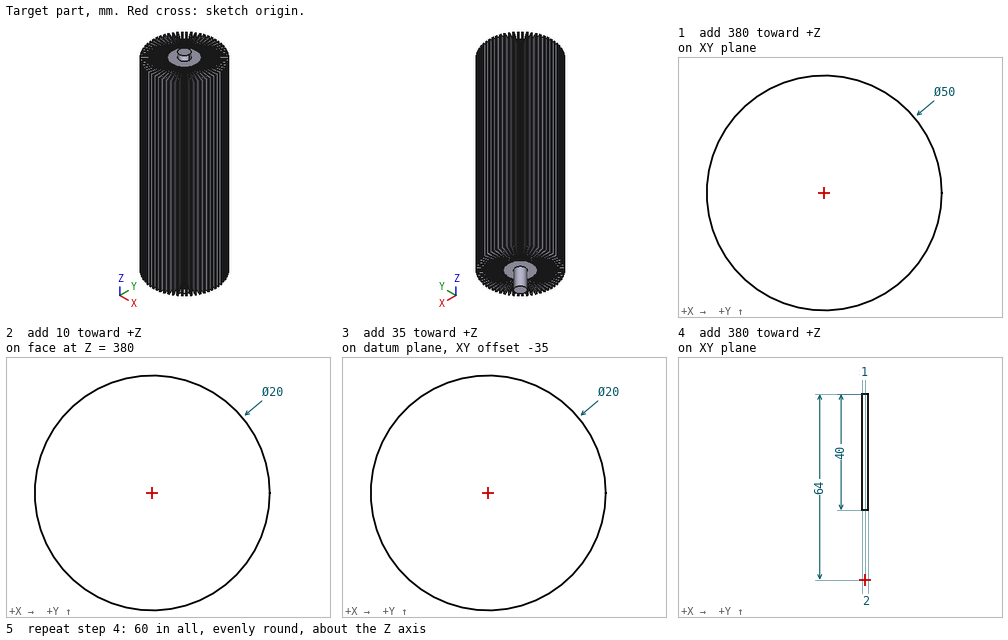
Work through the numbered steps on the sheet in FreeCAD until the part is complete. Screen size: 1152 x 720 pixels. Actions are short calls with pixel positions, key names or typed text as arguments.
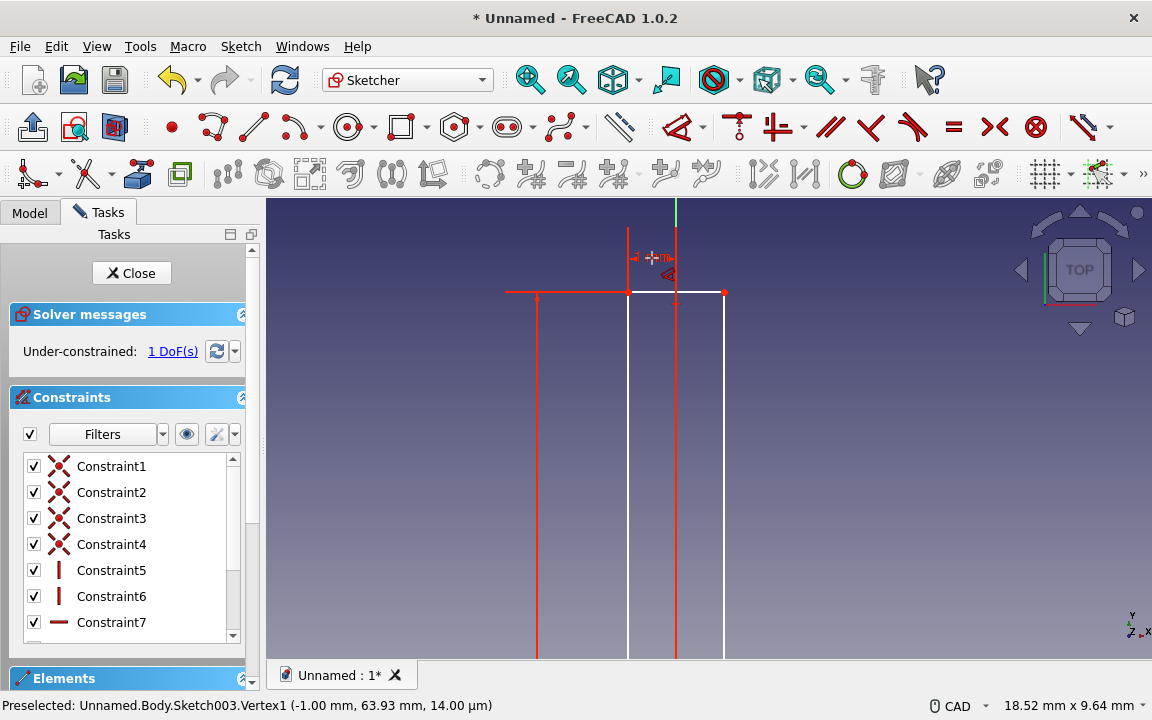
scroll(637, 290, down, 12)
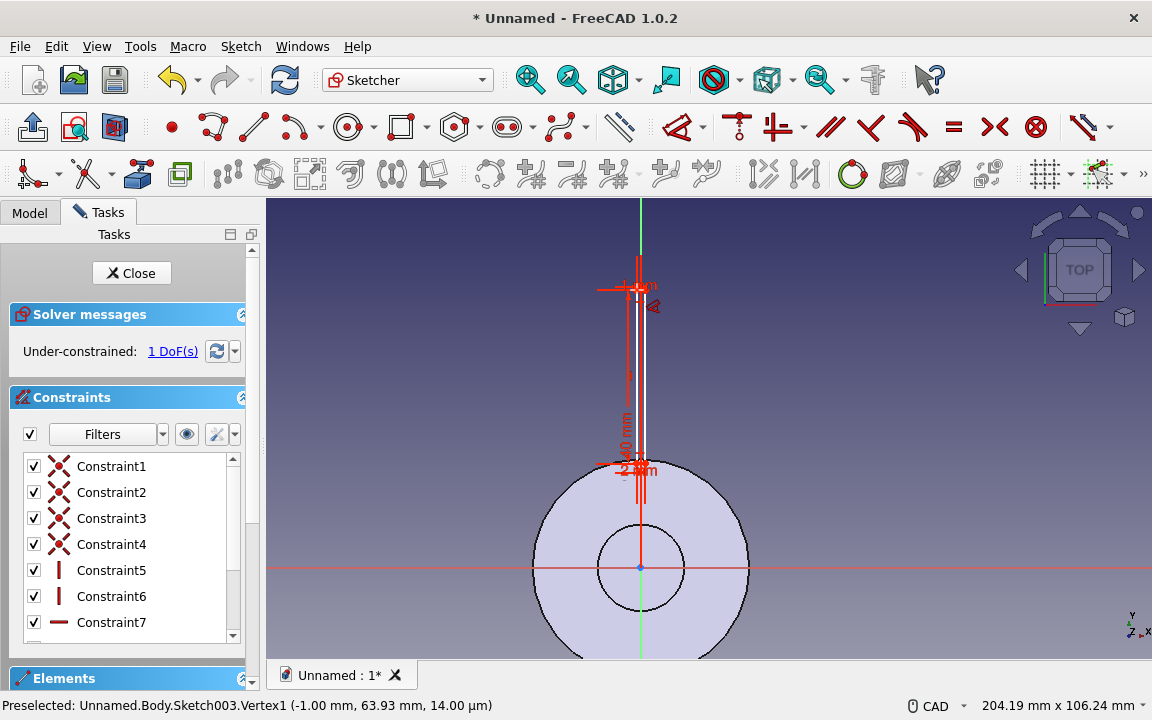
scroll(637, 290, up, 2)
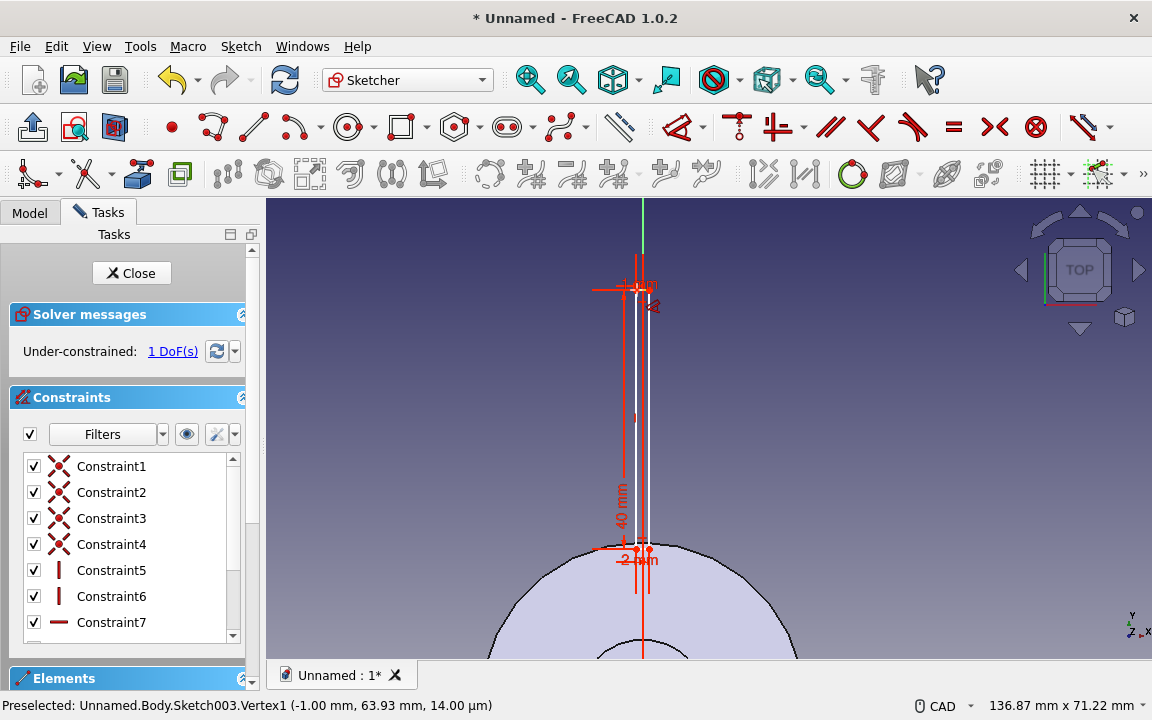
click(636, 290)
click(602, 461)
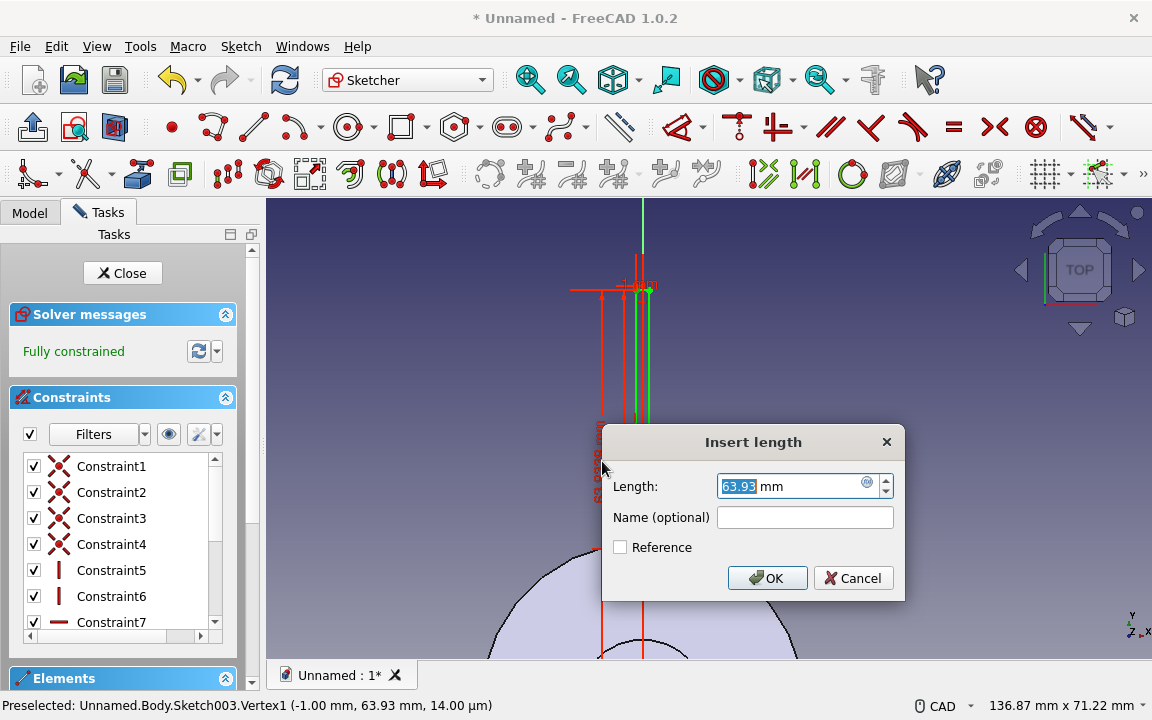
text(64)
key(Return)
key(Escape)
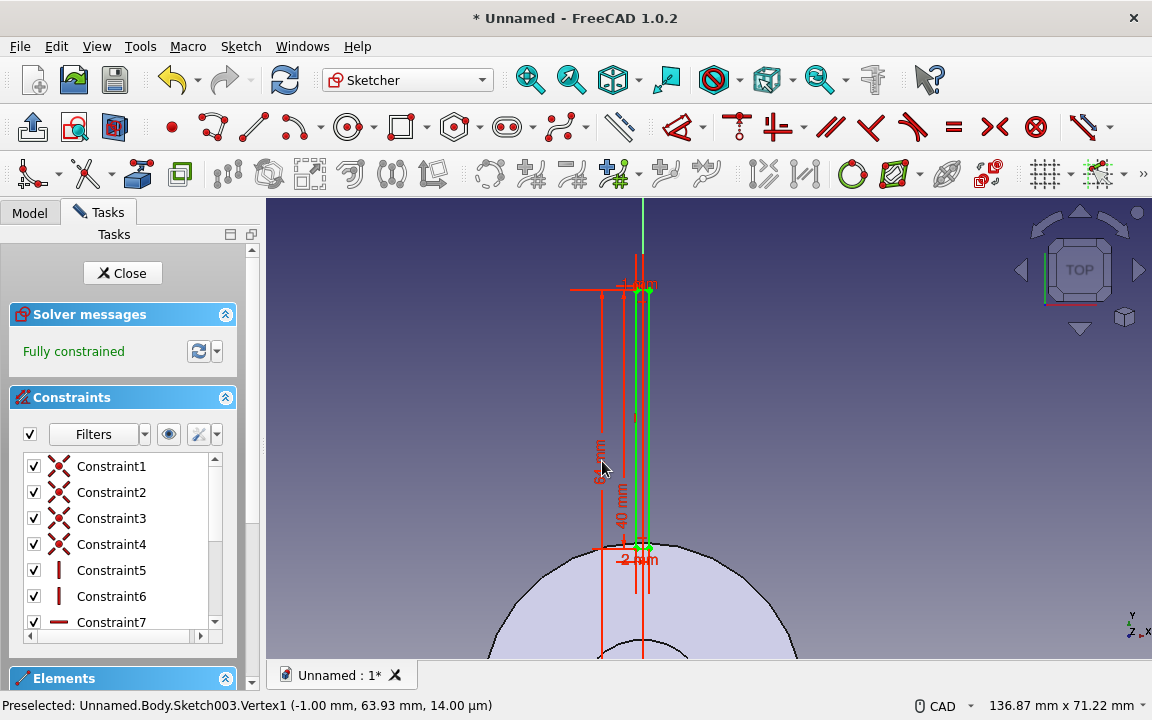
click(123, 273)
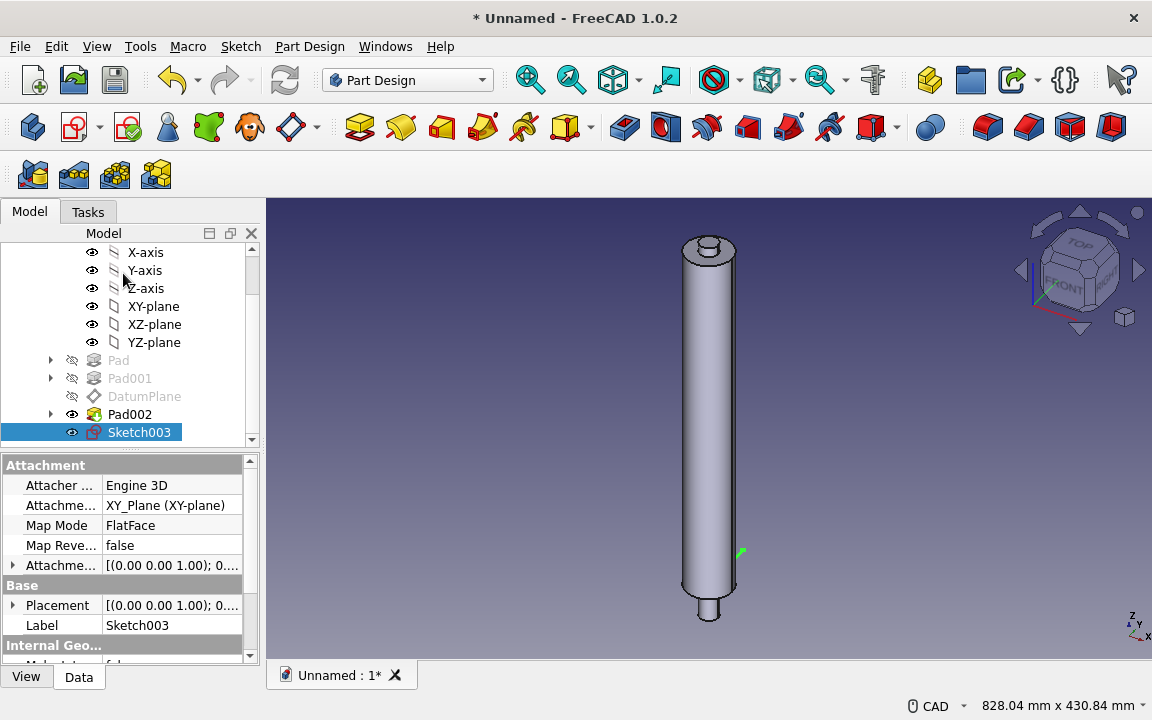
click(360, 128)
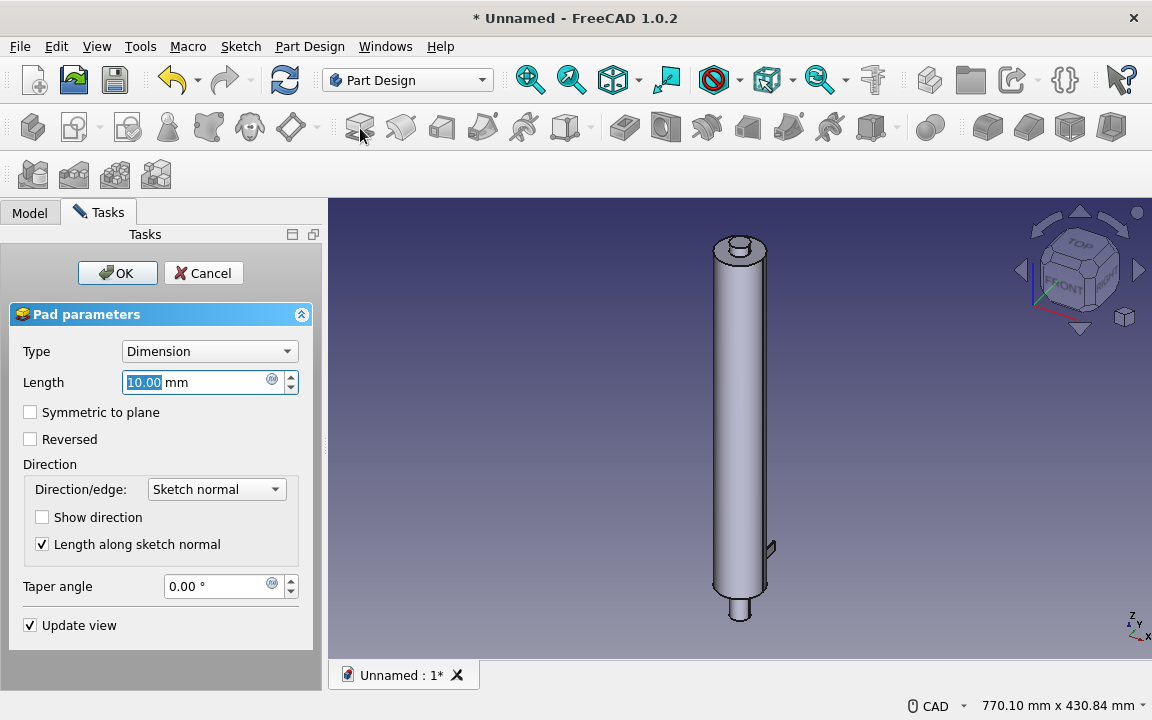
text(380)
key(Tab)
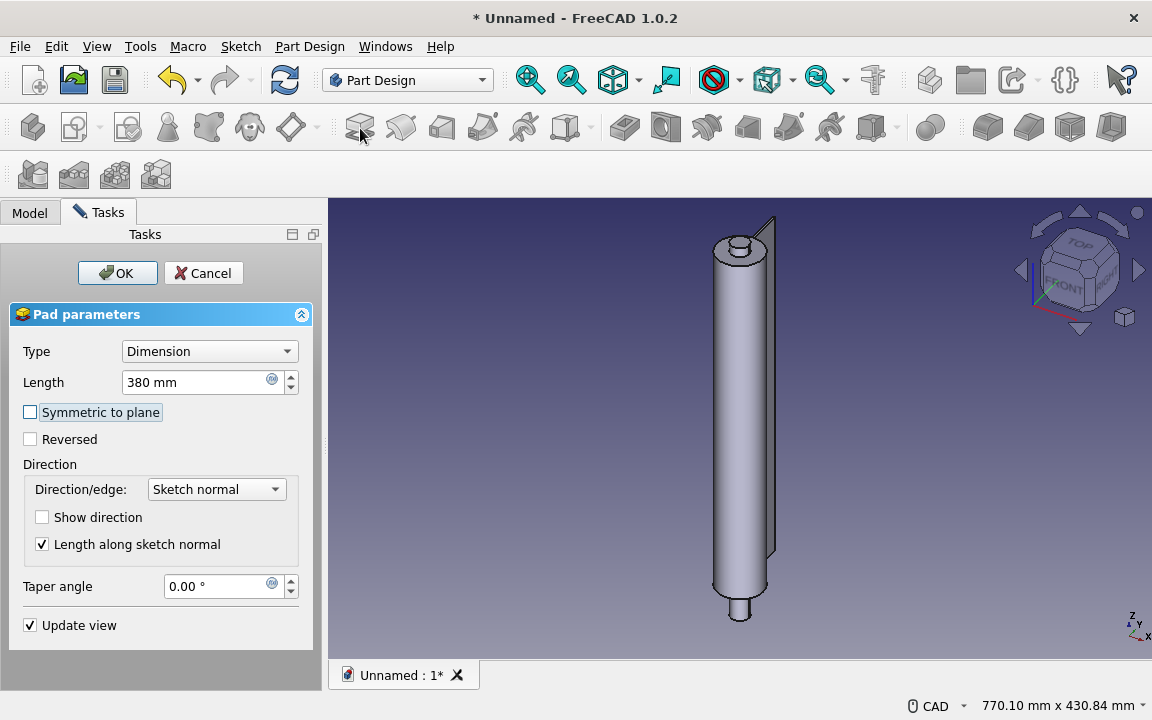
click(118, 273)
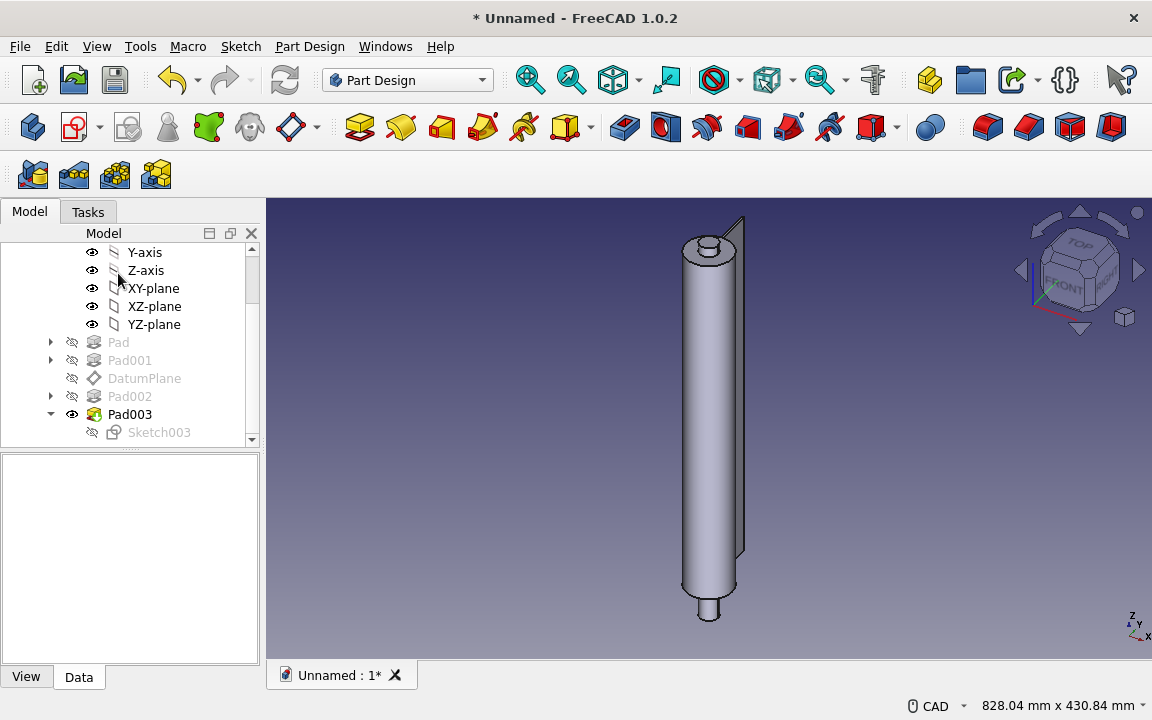
click(117, 414)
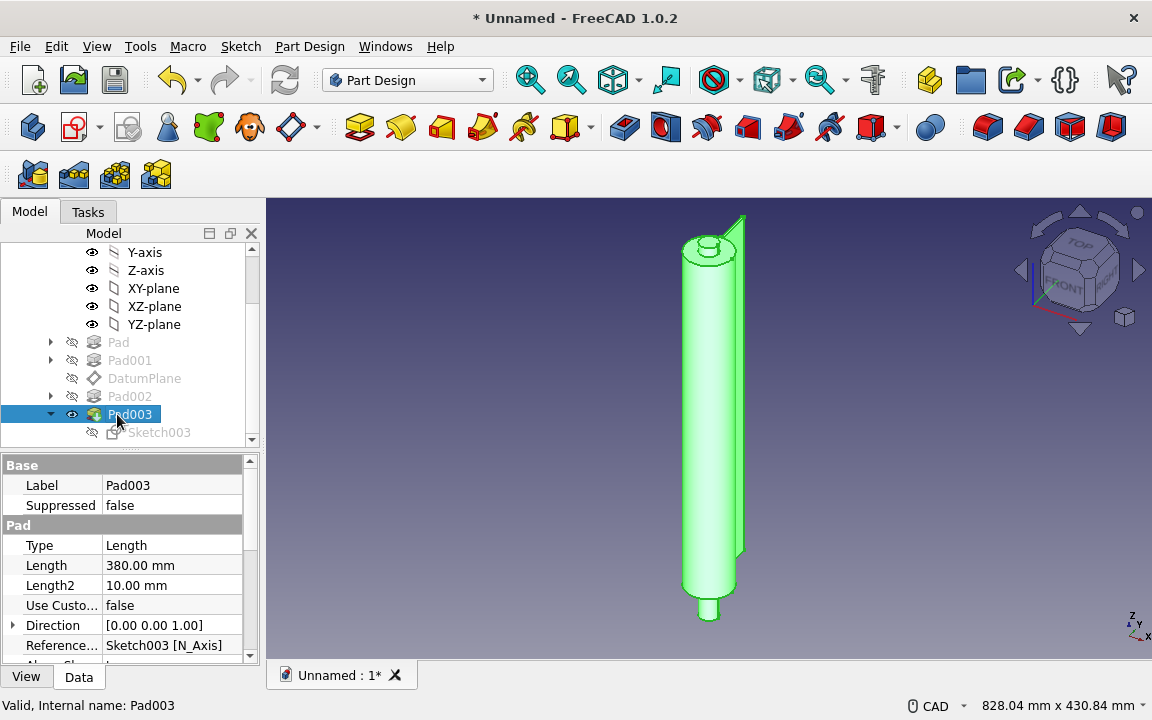
click(115, 174)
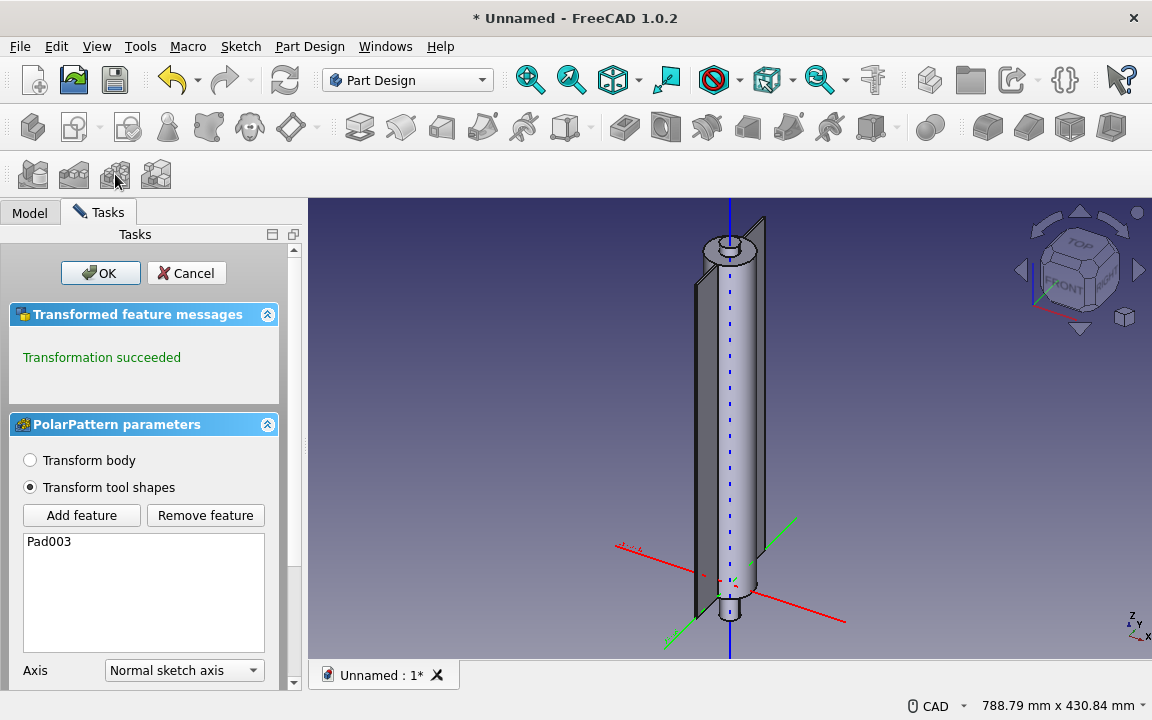
click(185, 670)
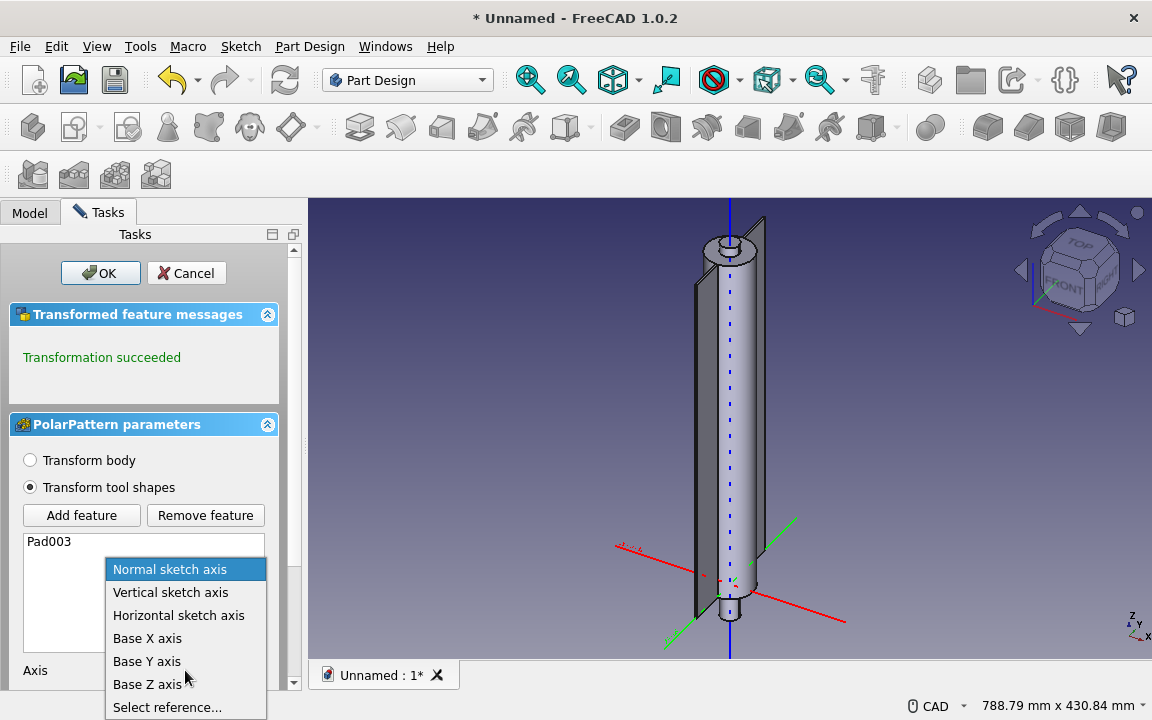
click(184, 684)